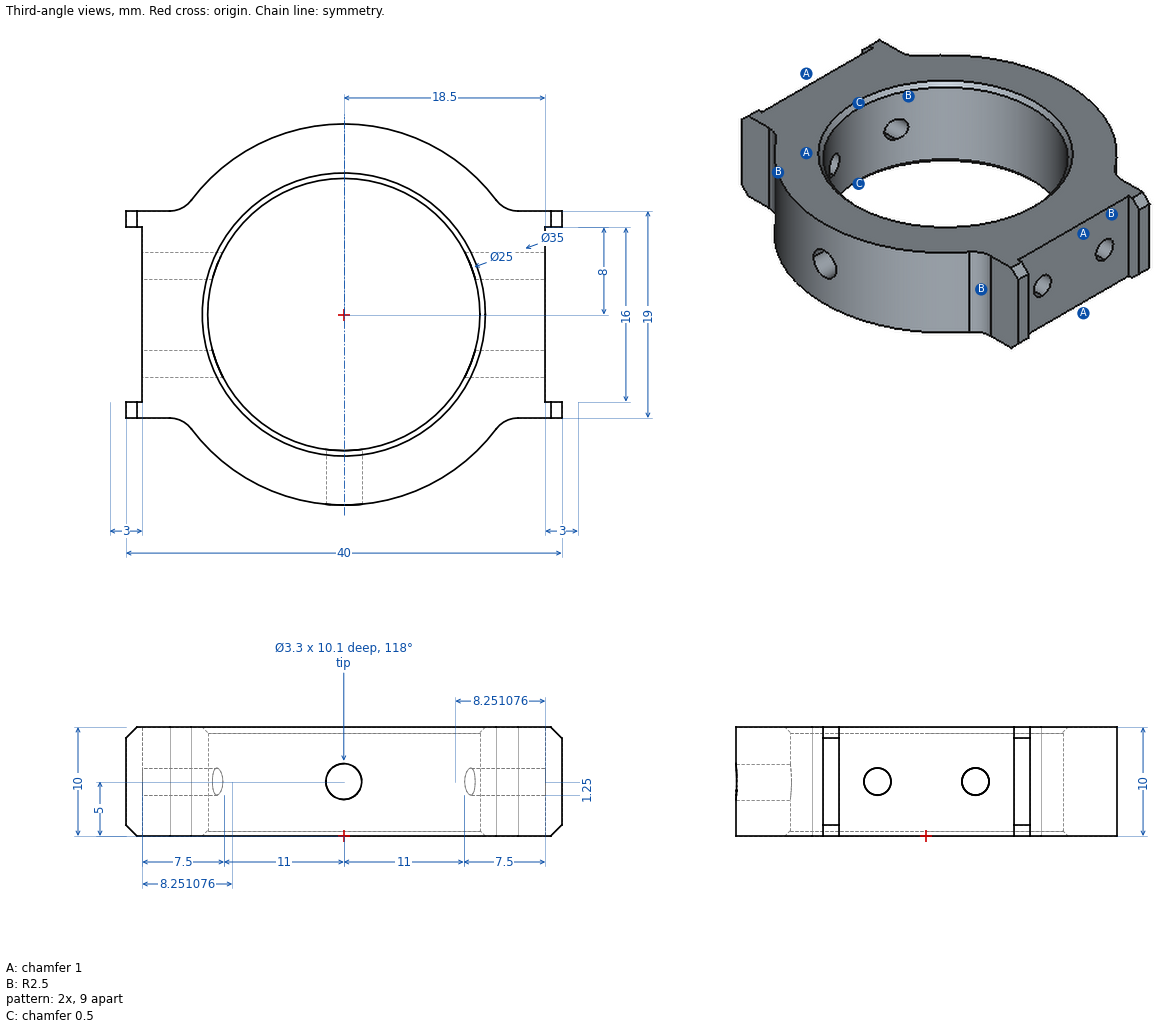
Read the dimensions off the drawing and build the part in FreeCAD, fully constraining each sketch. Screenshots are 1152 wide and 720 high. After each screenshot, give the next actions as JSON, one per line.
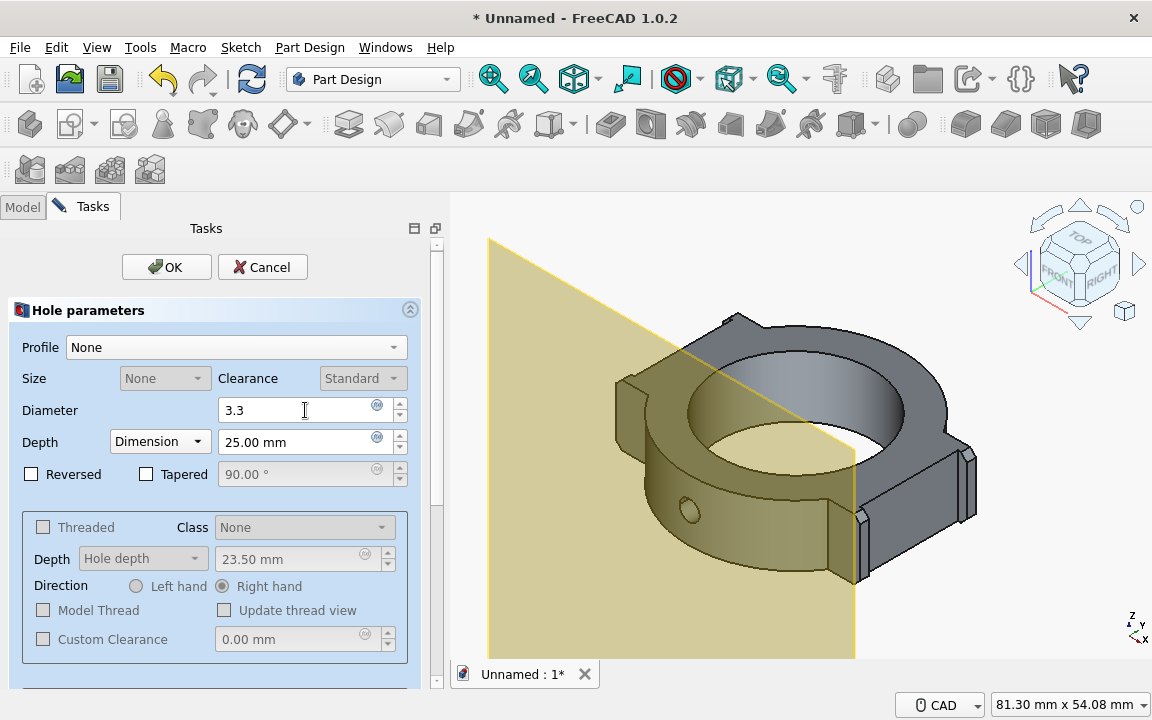
{"action": "triple_click", "coordinate": [305, 442]}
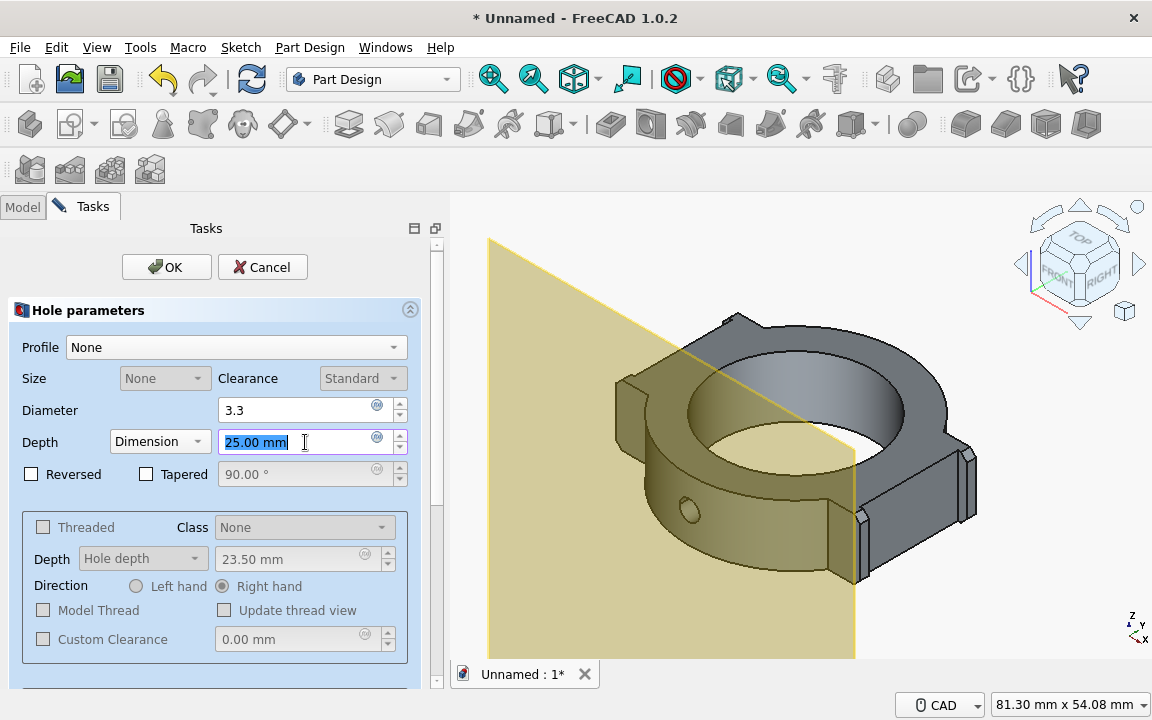
{"action": "type", "text": "10.1"}
{"action": "key", "text": "Tab"}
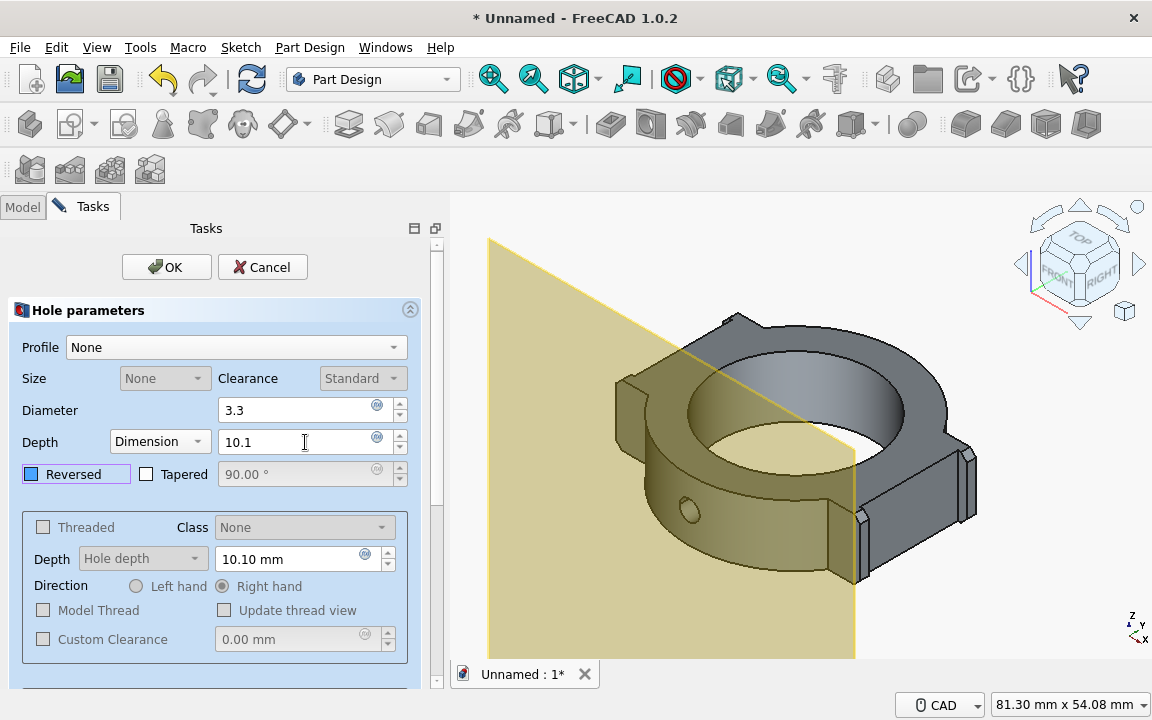
{"action": "left_click", "coordinate": [167, 267]}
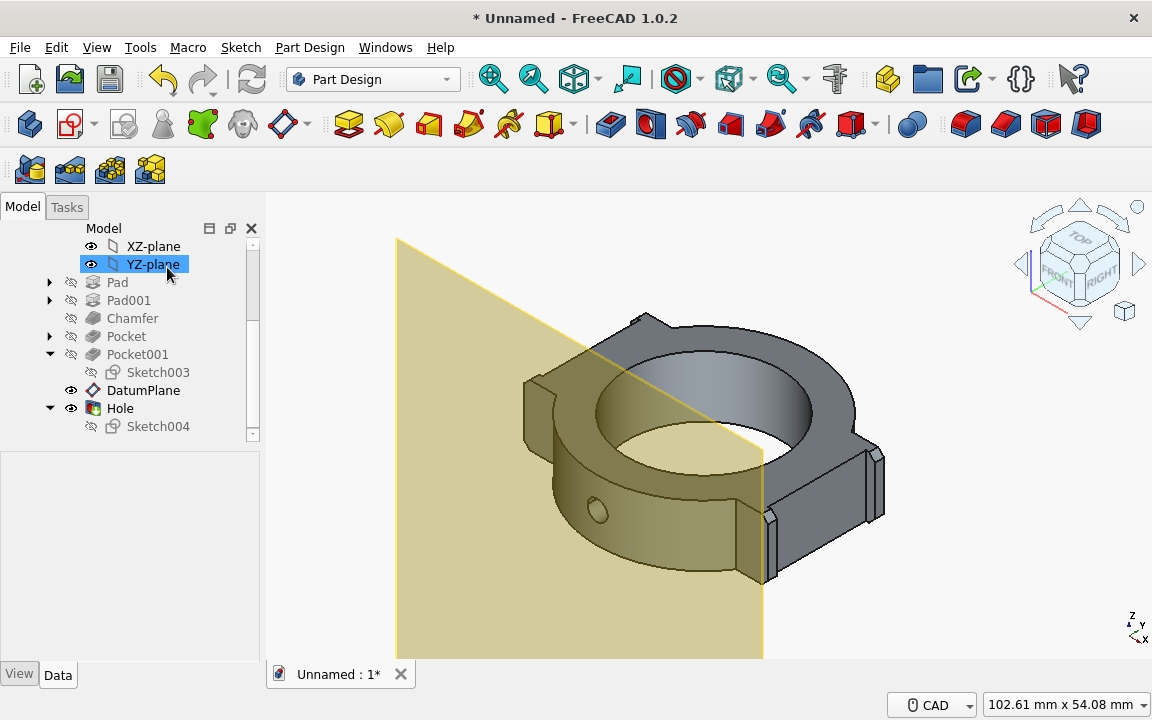
{"action": "left_click", "coordinate": [116, 390]}
{"action": "key", "text": "space"}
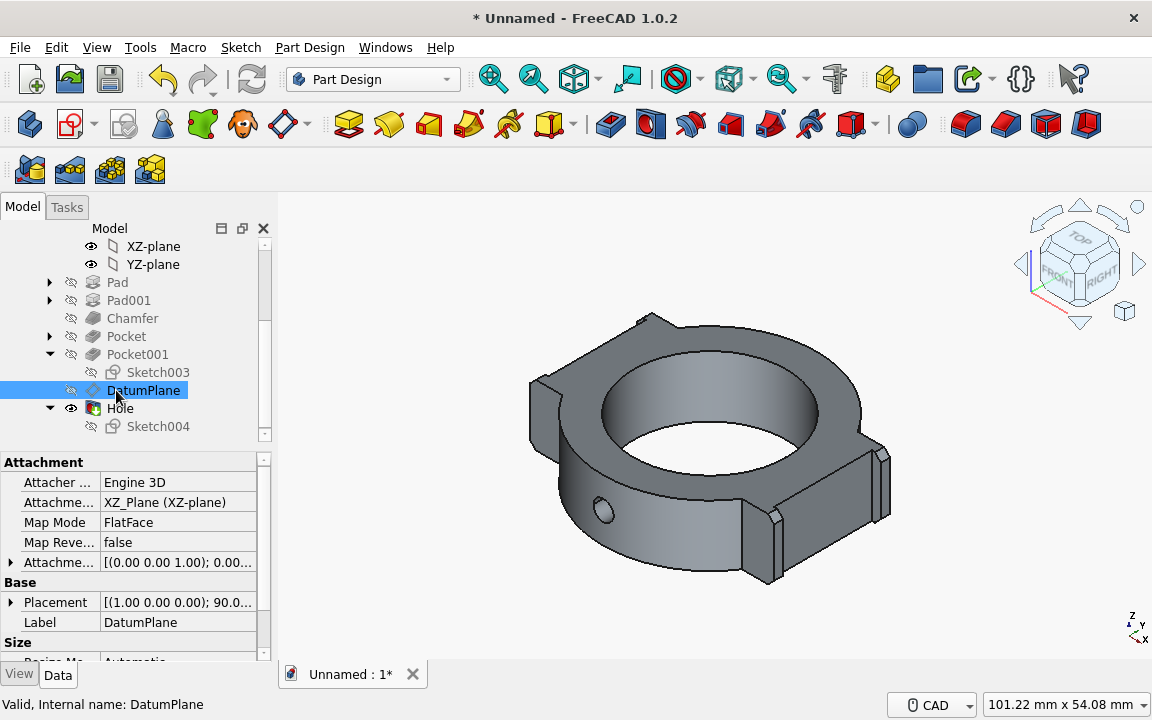
{"action": "key", "text": "2"}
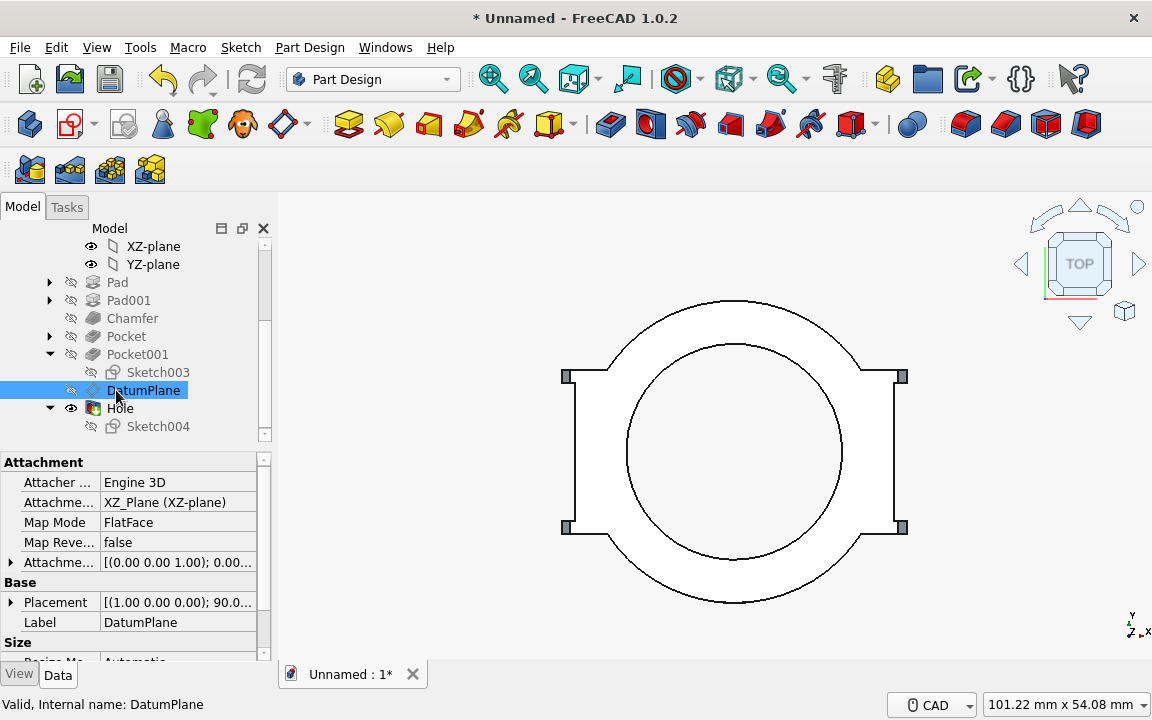
{"action": "key", "text": "0"}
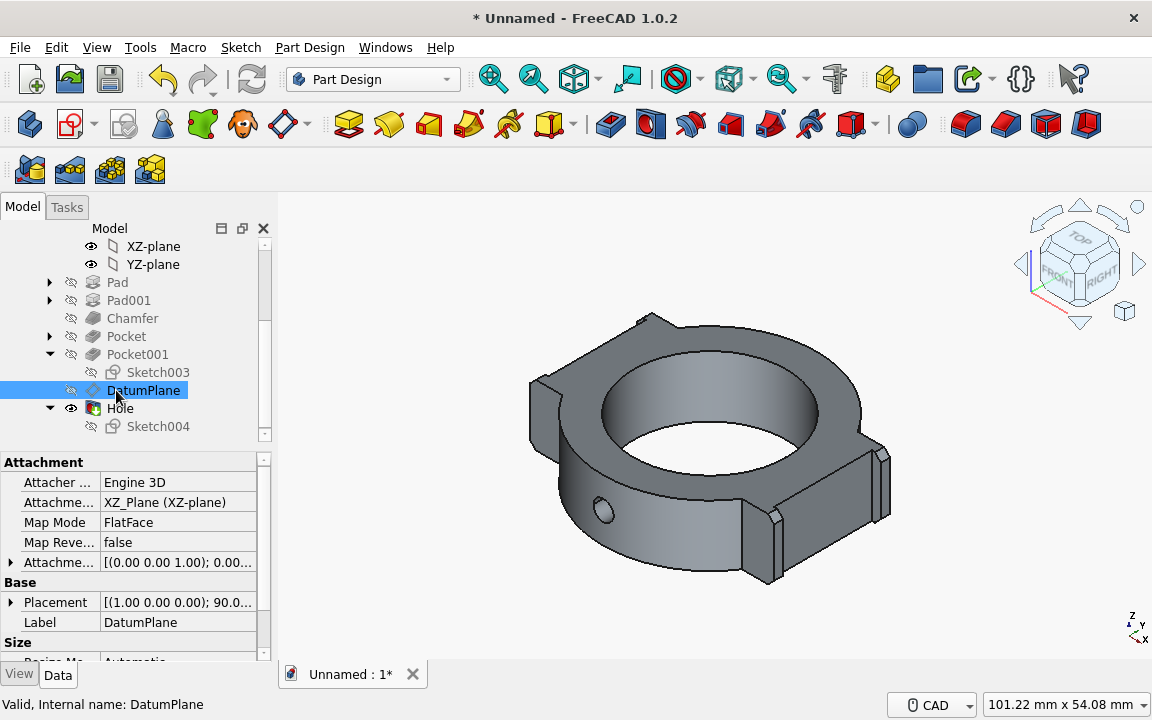
{"action": "key", "text": "1"}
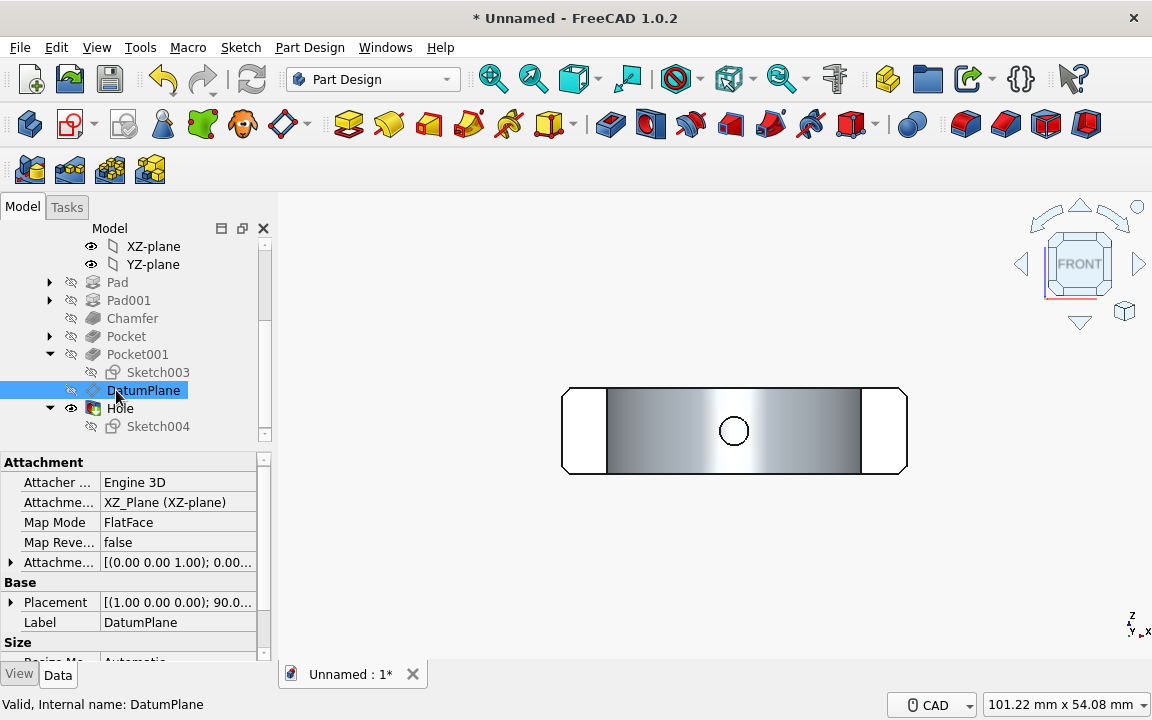
{"action": "left_click", "coordinate": [494, 80]}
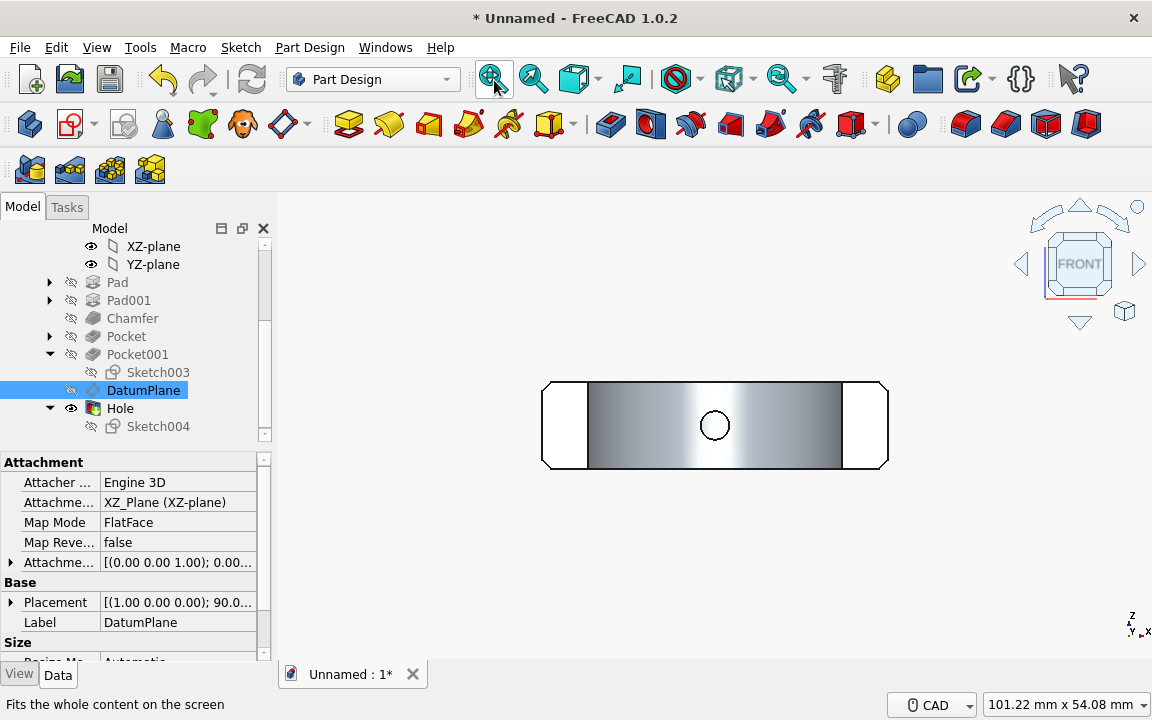
{"action": "key", "text": "3"}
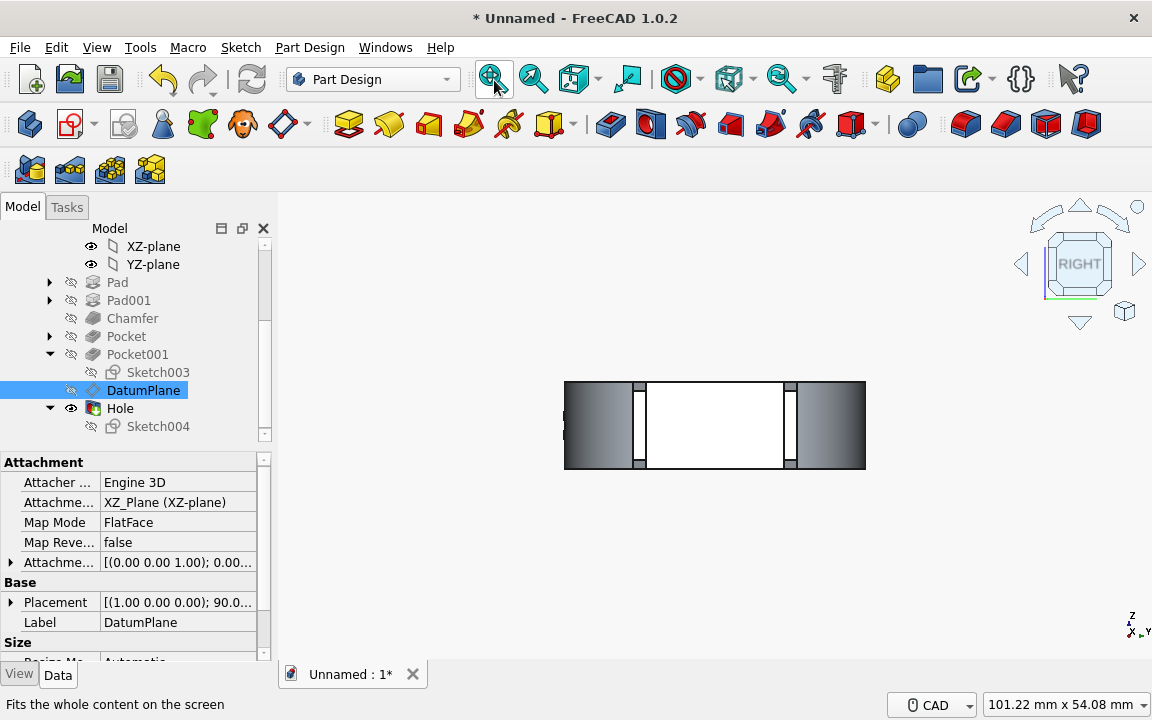
{"action": "left_click", "coordinate": [494, 80]}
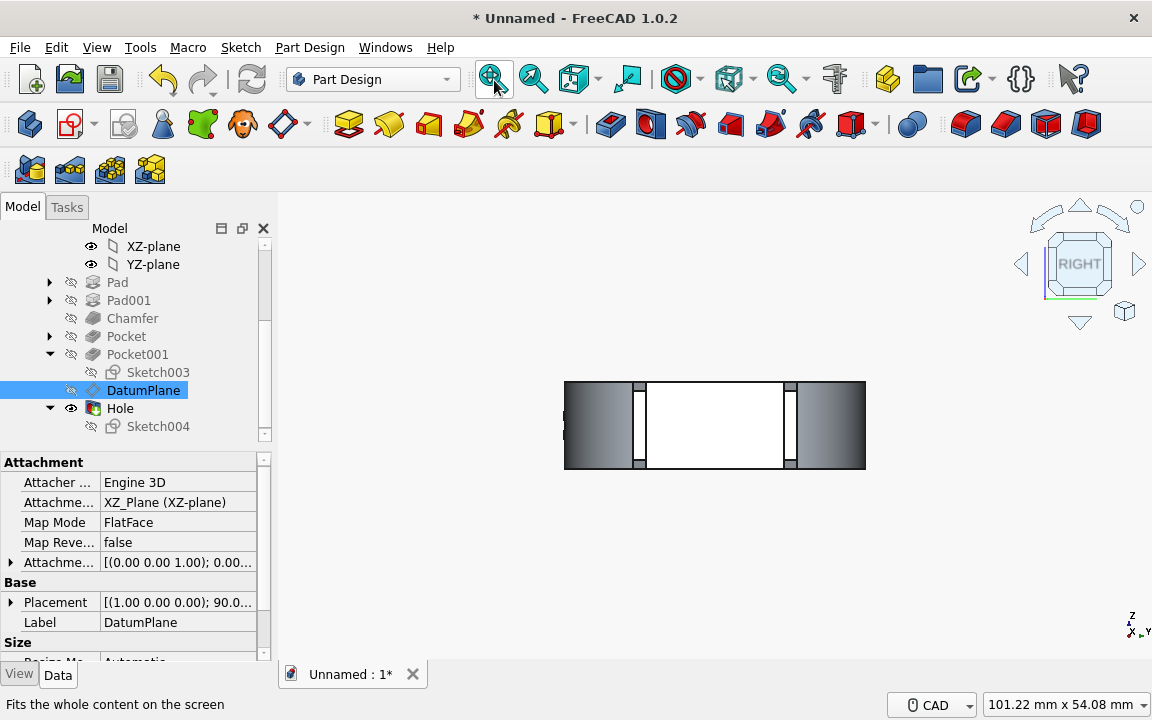
{"action": "key", "text": "5"}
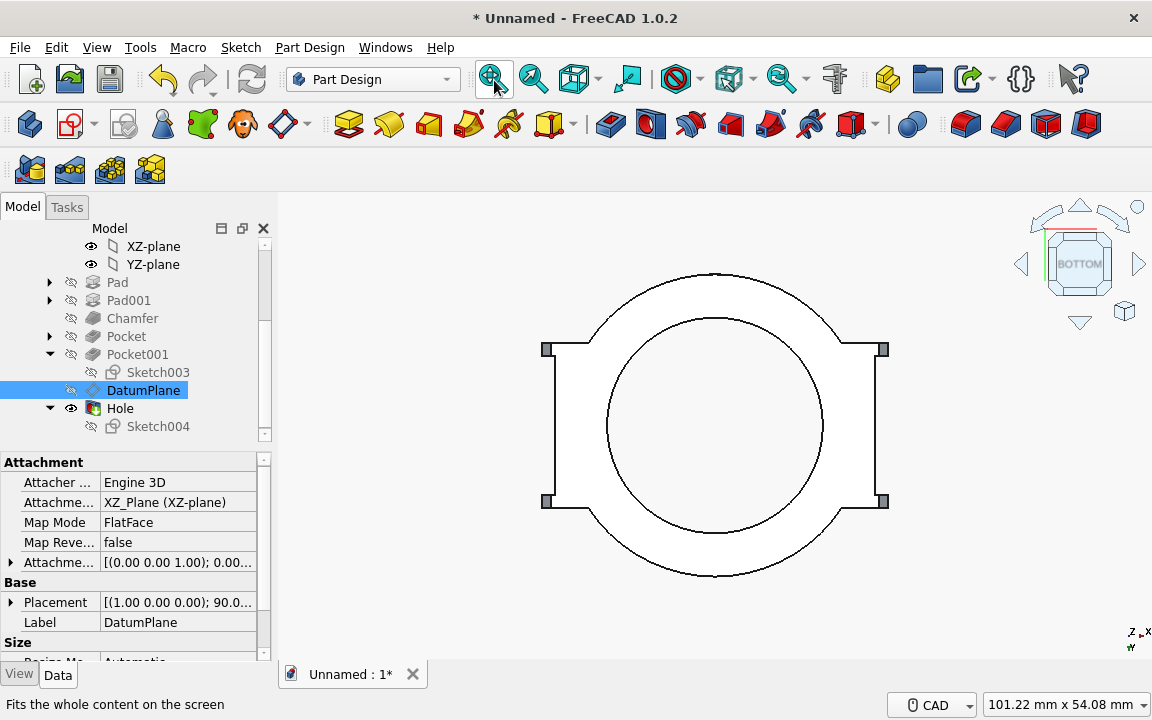
{"action": "key", "text": "4"}